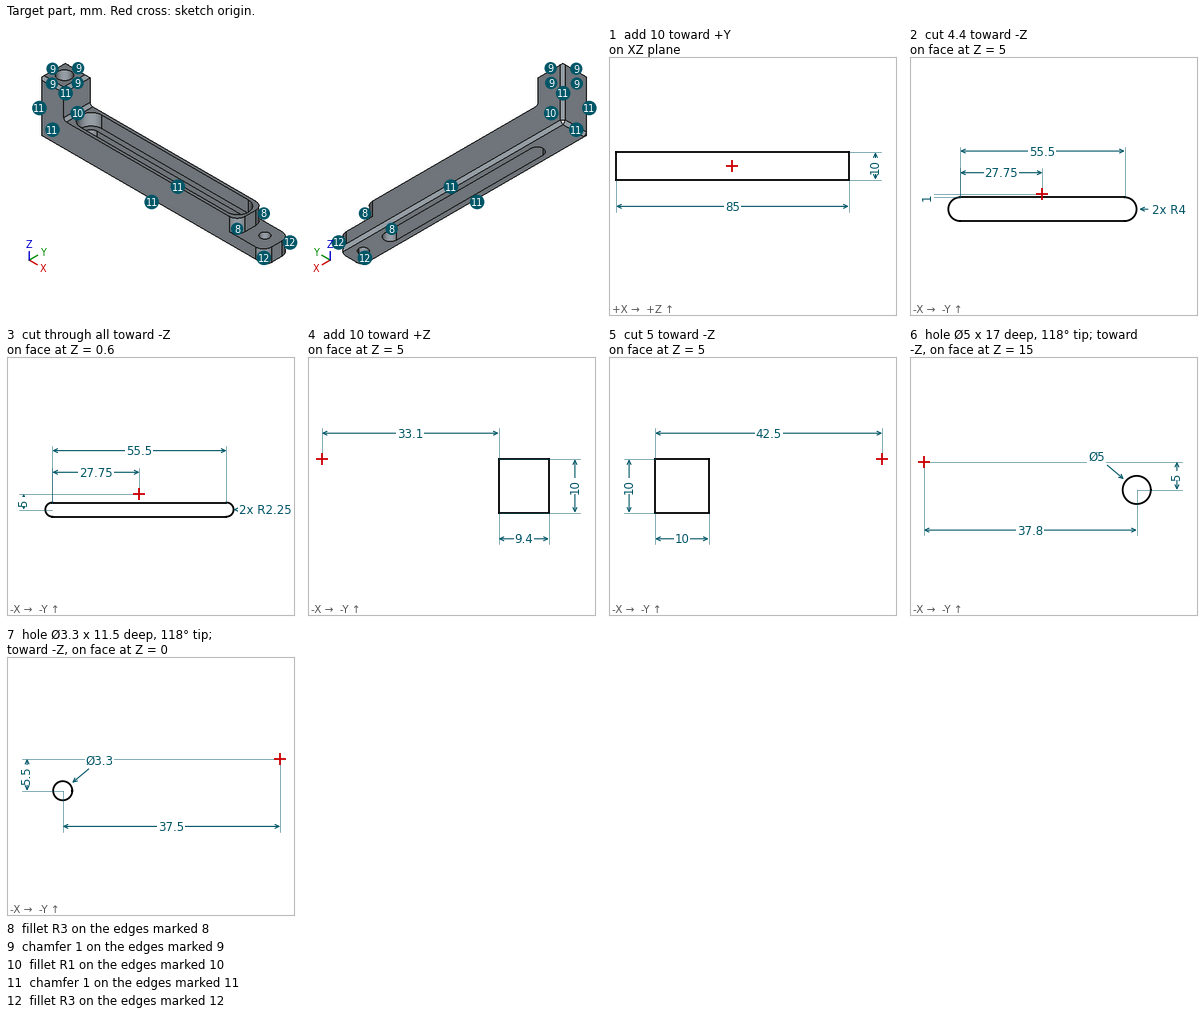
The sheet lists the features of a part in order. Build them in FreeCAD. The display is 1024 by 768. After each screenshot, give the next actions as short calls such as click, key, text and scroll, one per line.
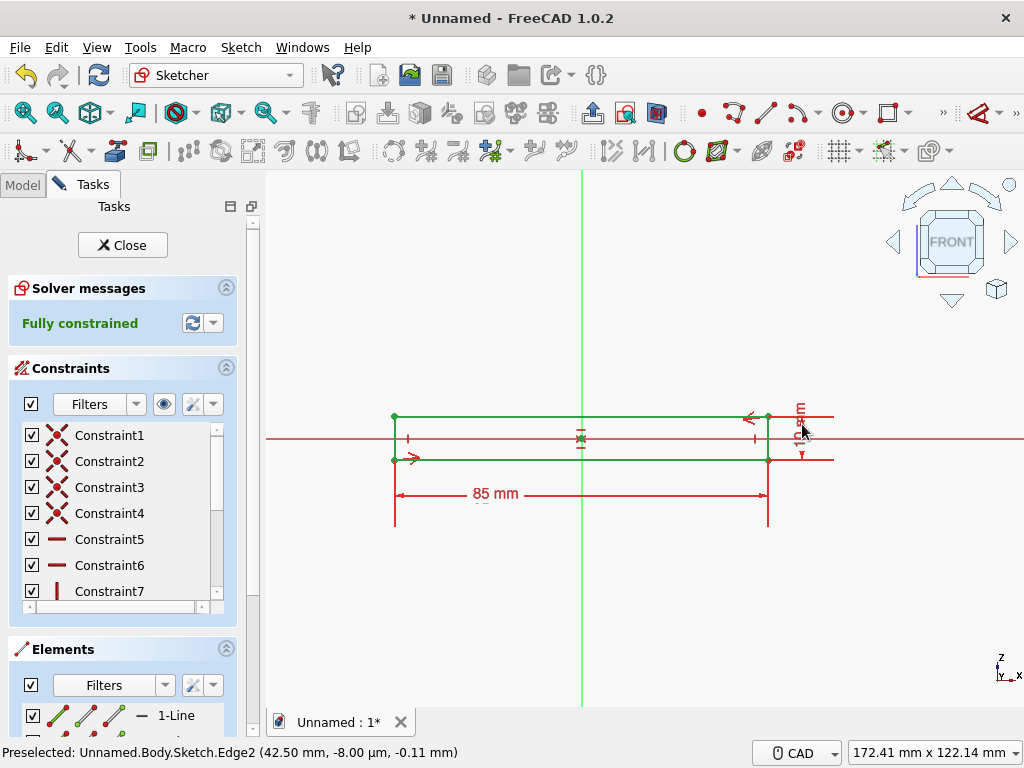
click(123, 245)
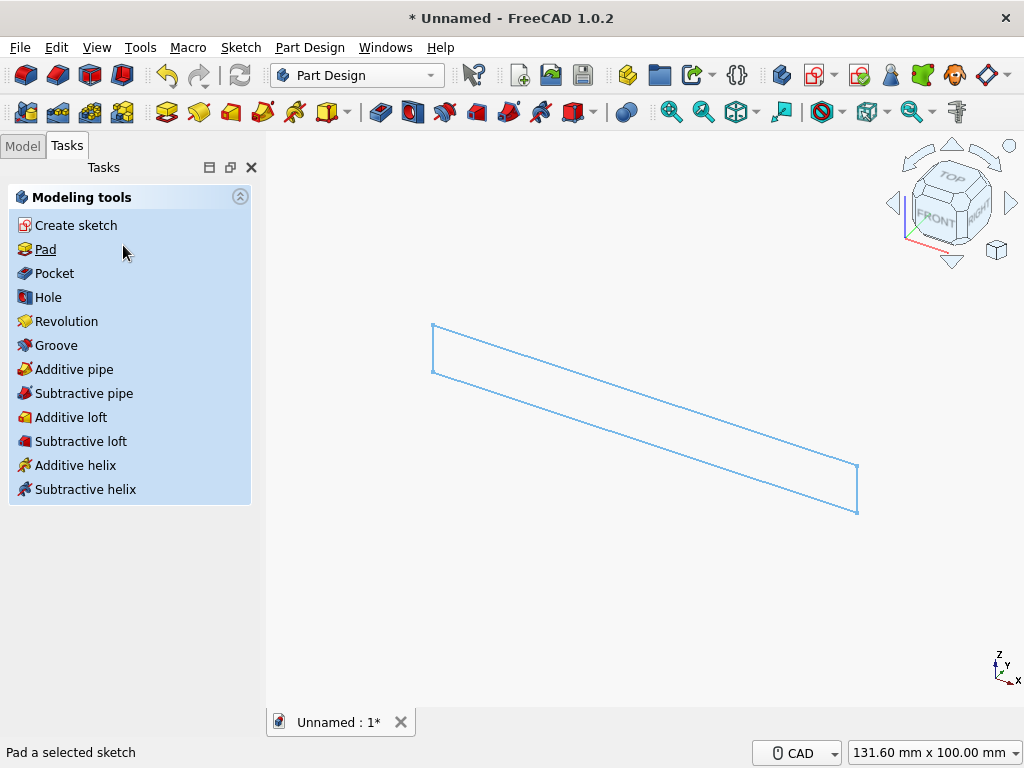
click(168, 112)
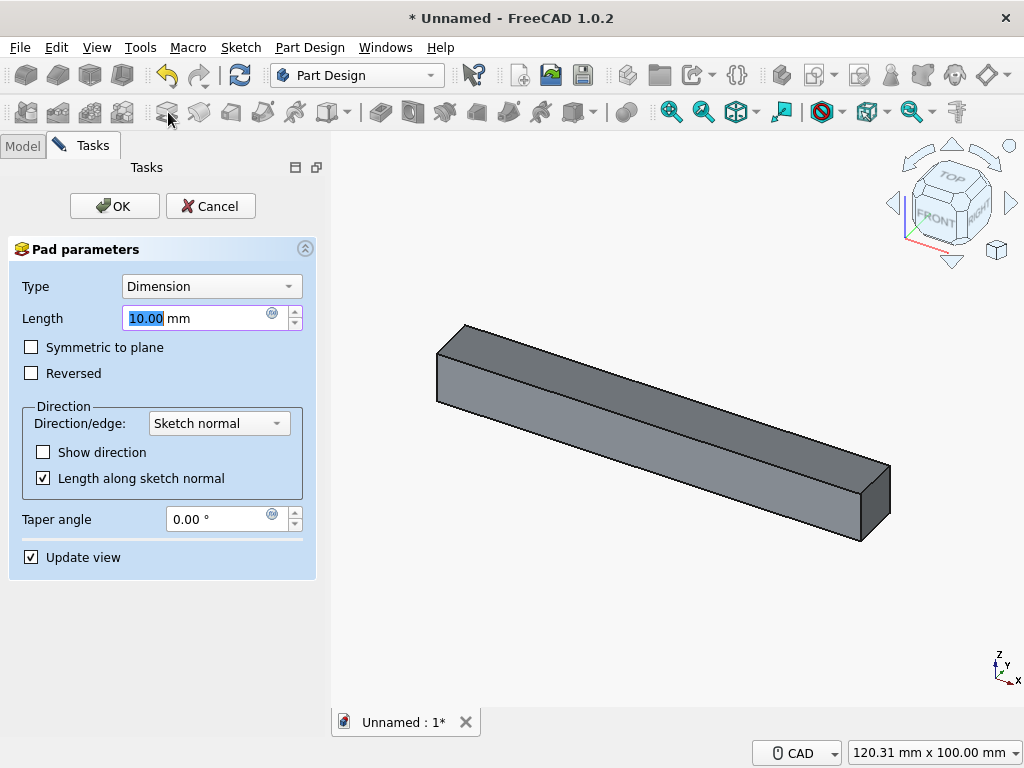
text(10)
key(Tab)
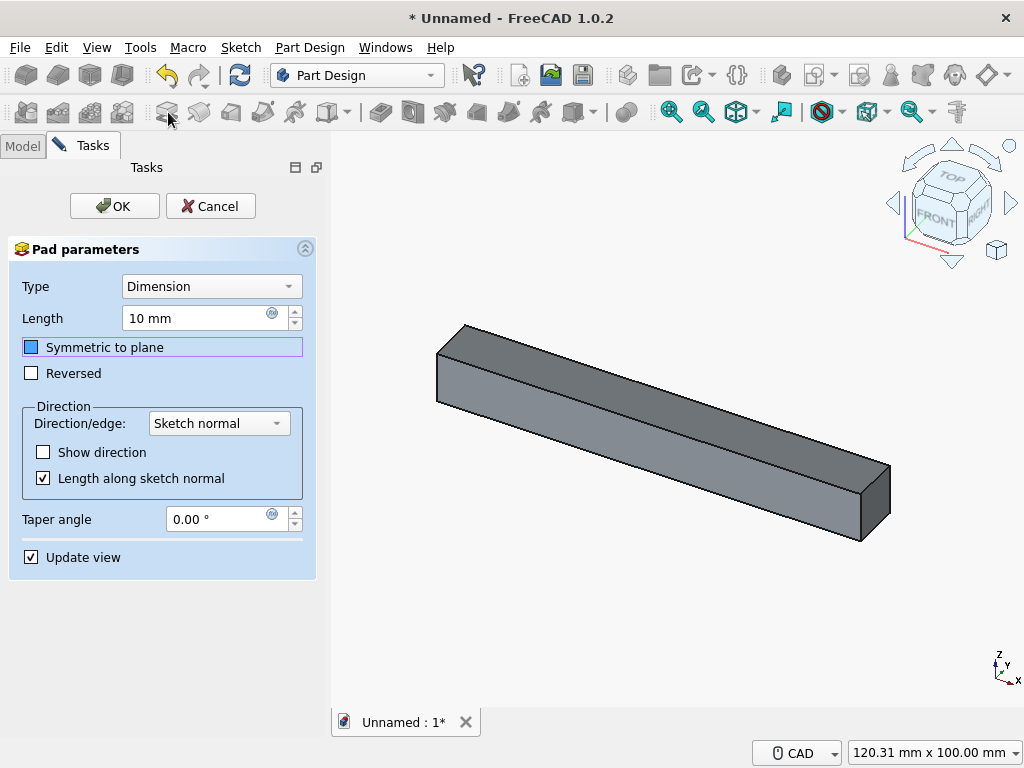
click(30, 373)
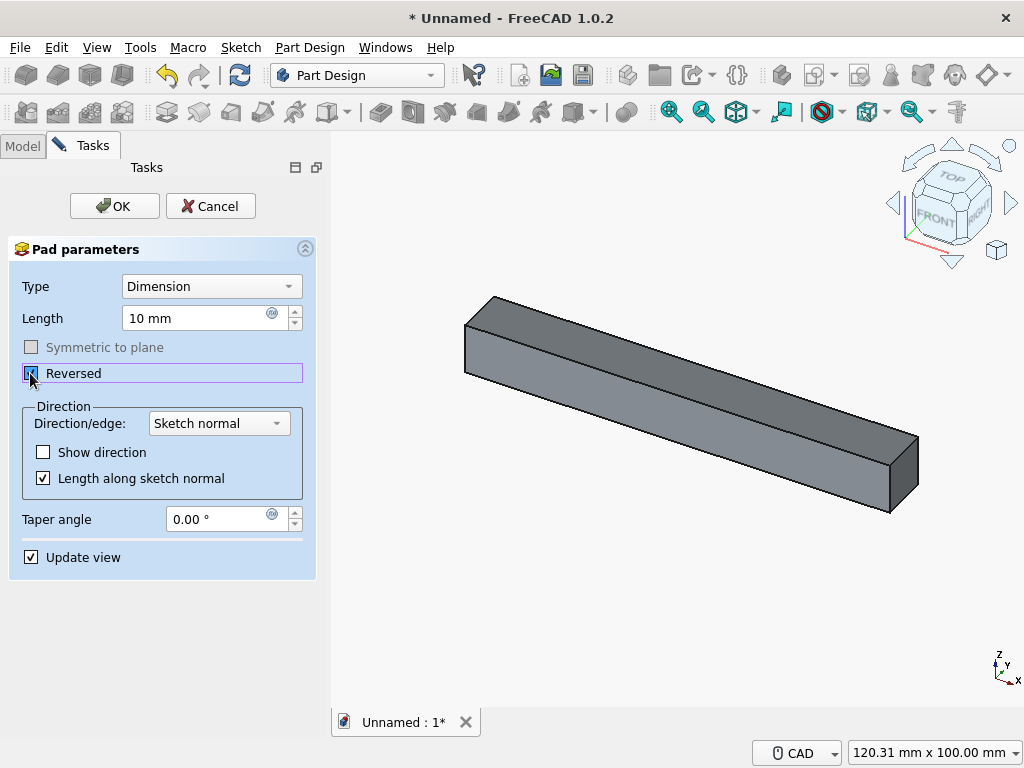
click(115, 206)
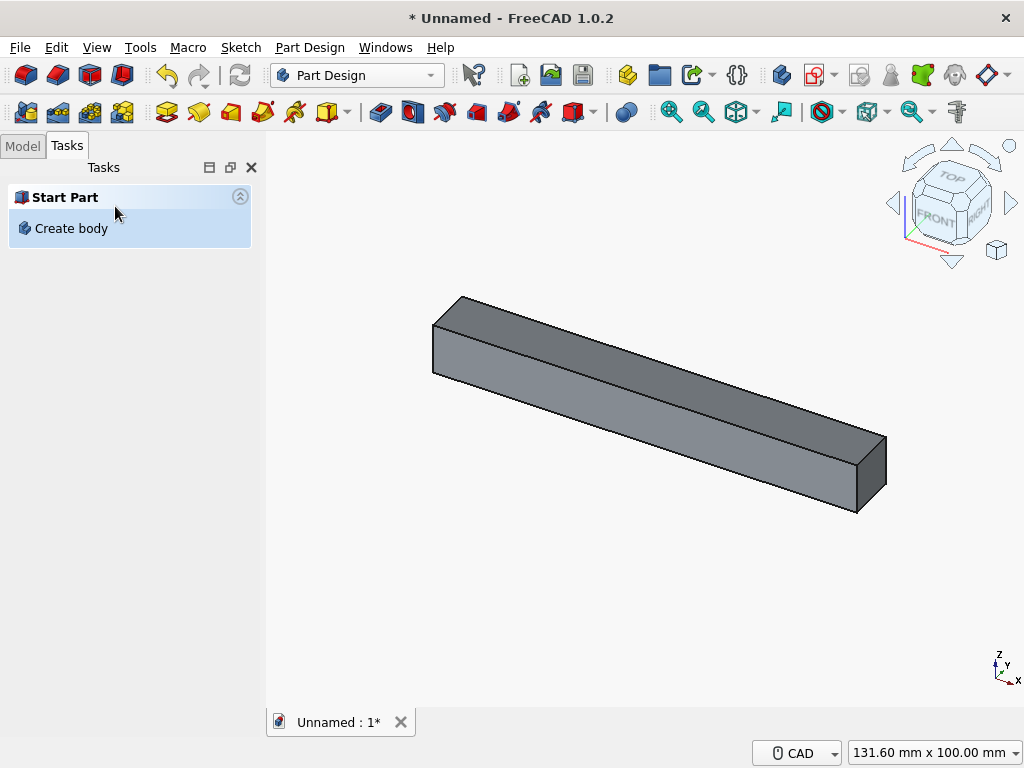
click(841, 440)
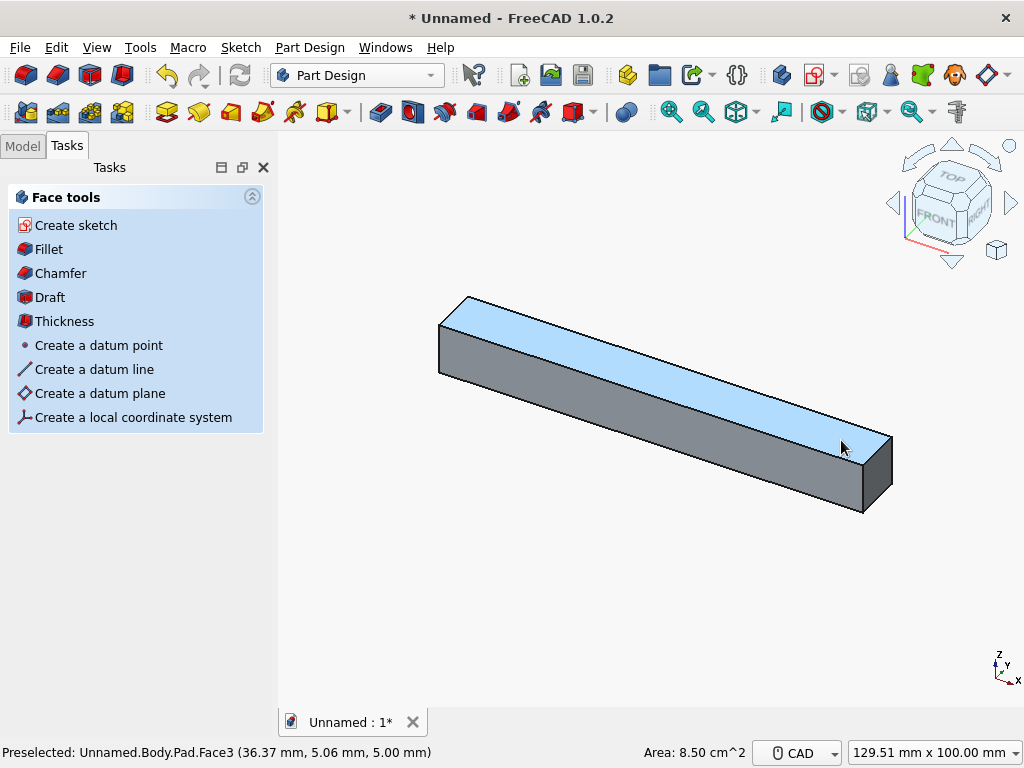
click(814, 76)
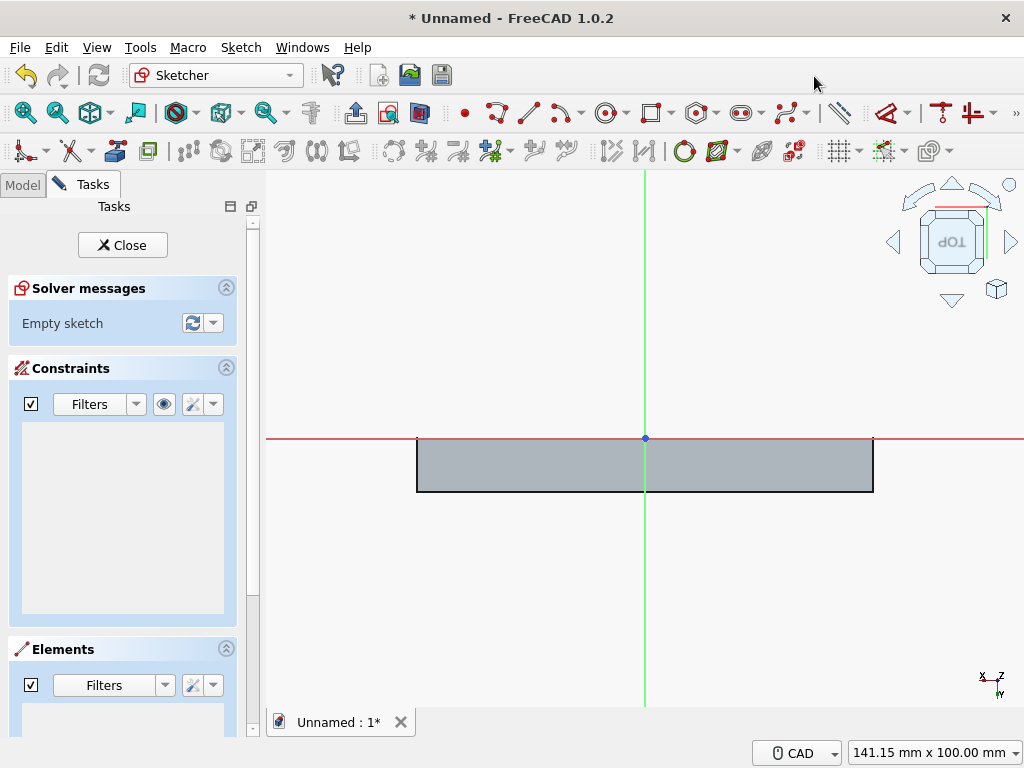
click(742, 114)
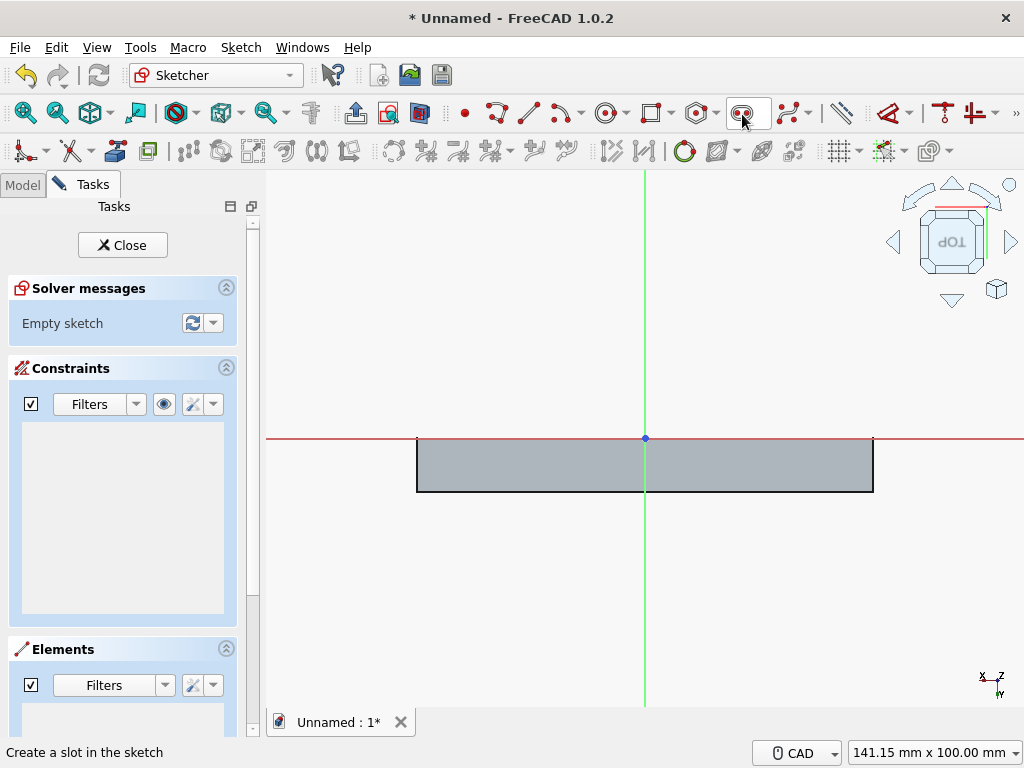
click(496, 465)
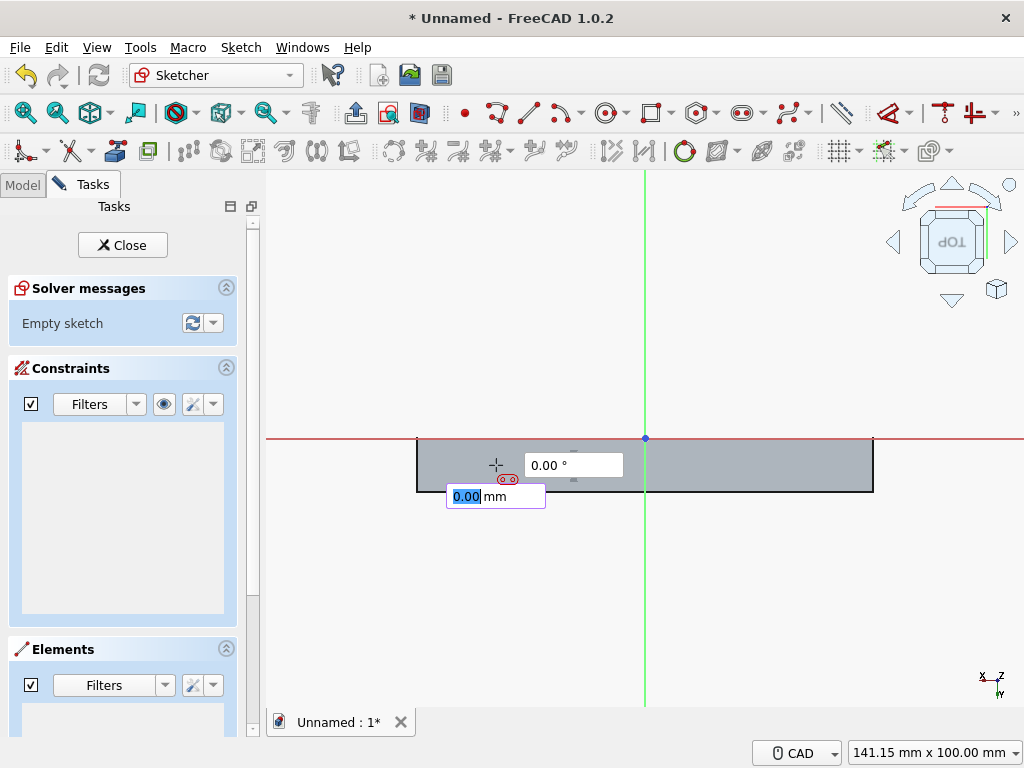
click(794, 465)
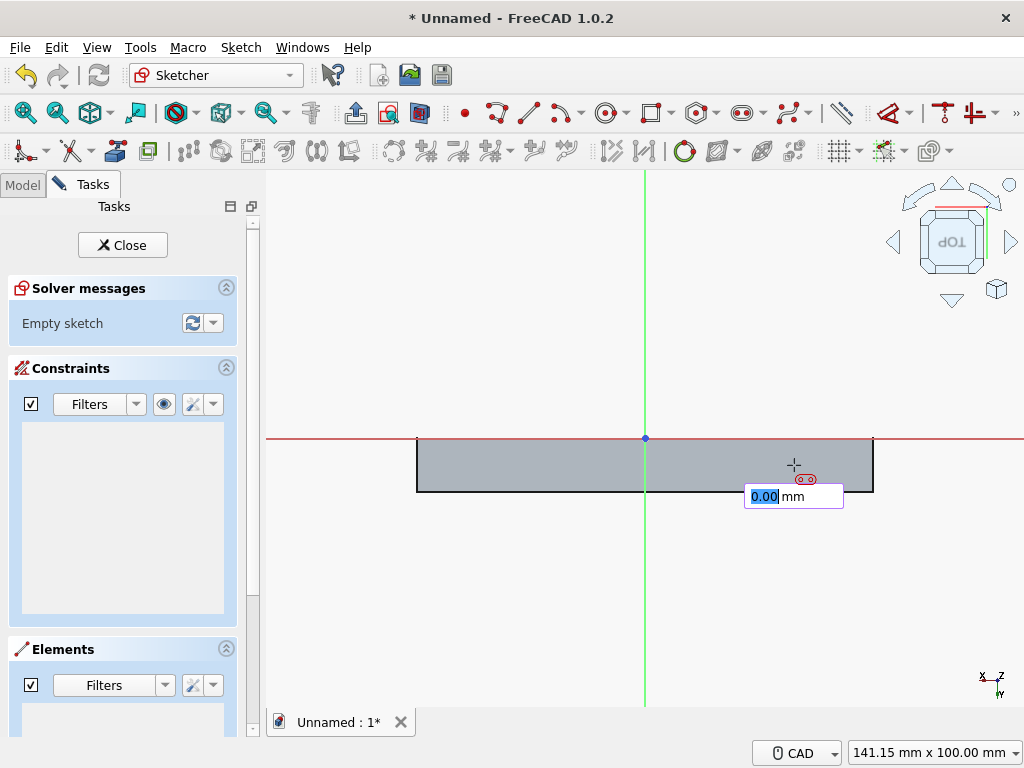
click(600, 487)
key(Escape)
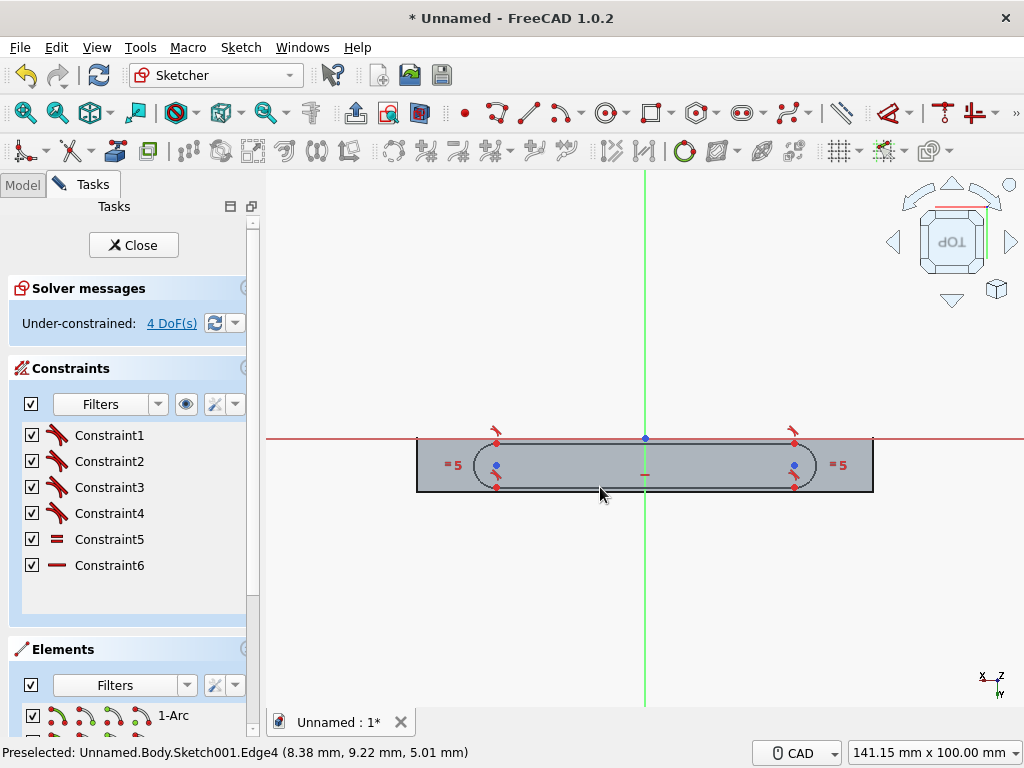
key(d)